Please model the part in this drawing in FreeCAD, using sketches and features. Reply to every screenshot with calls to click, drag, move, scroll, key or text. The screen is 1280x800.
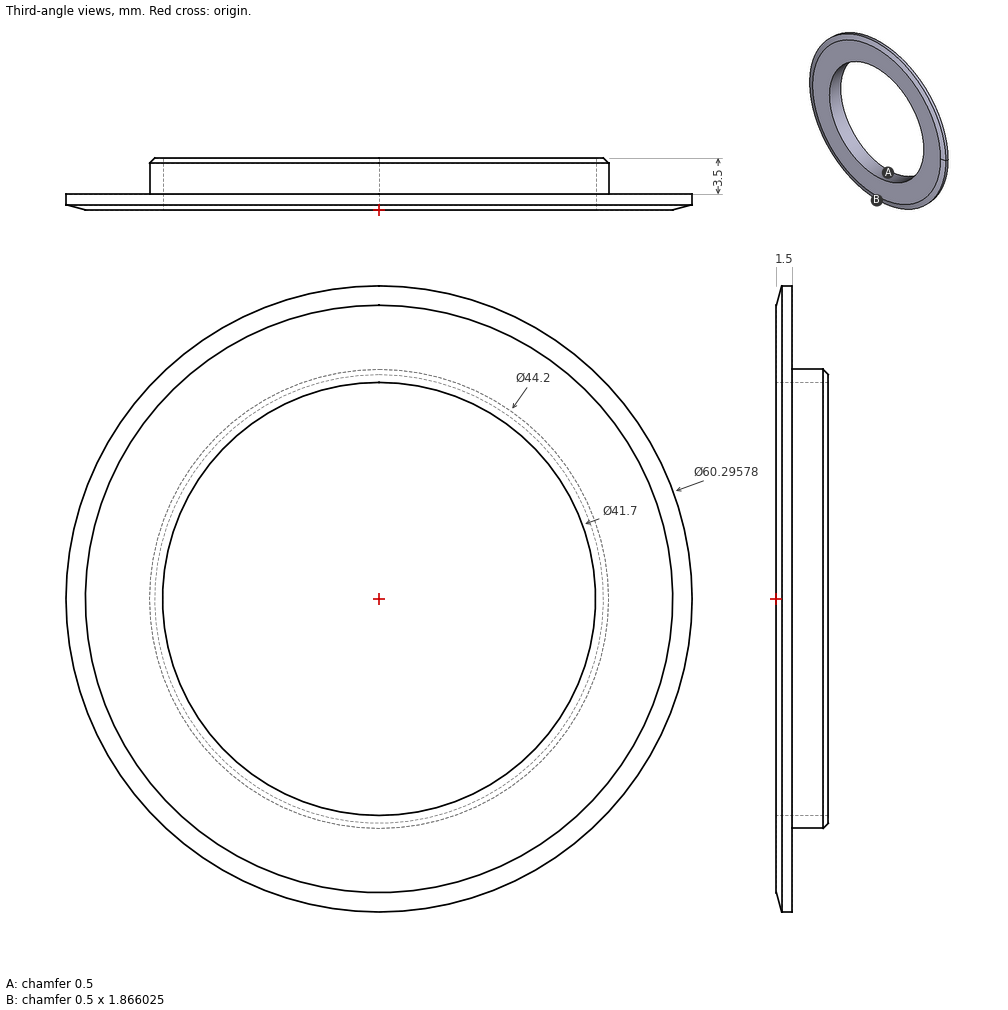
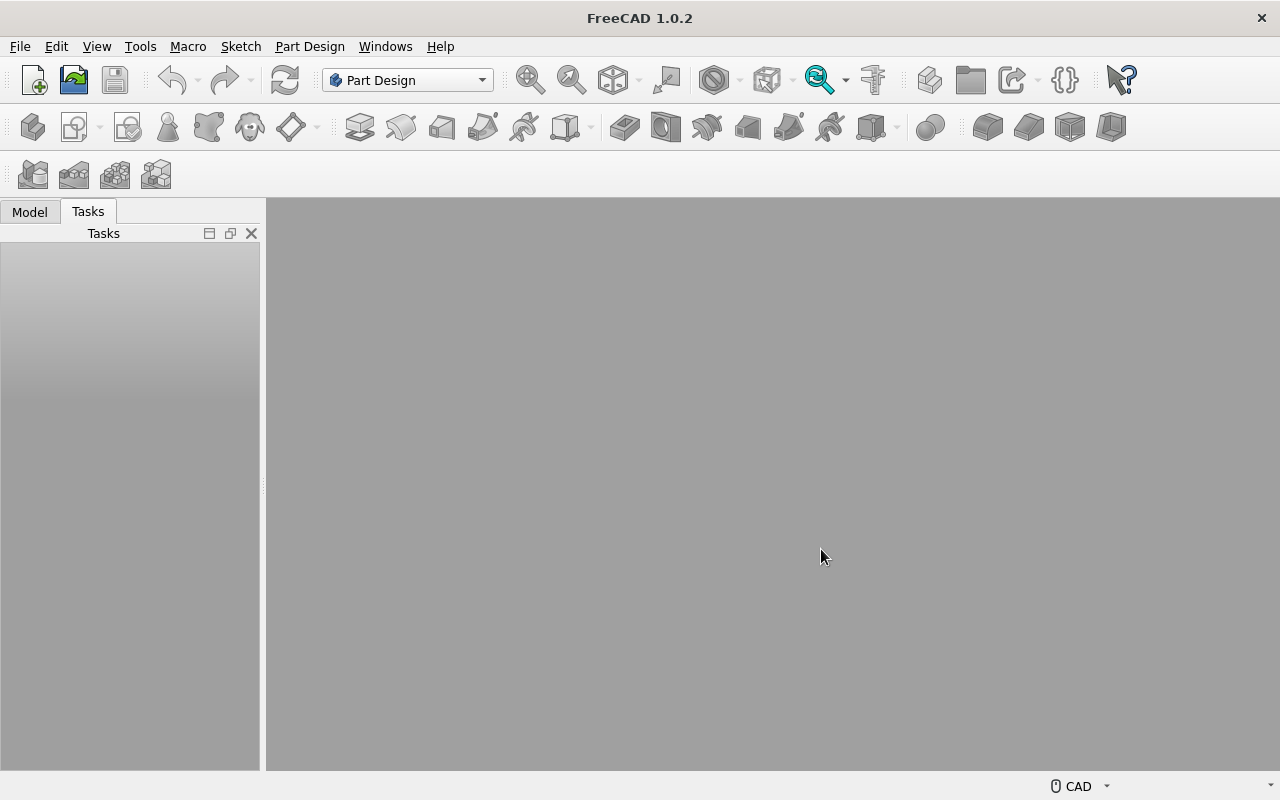
key(ctrl+n)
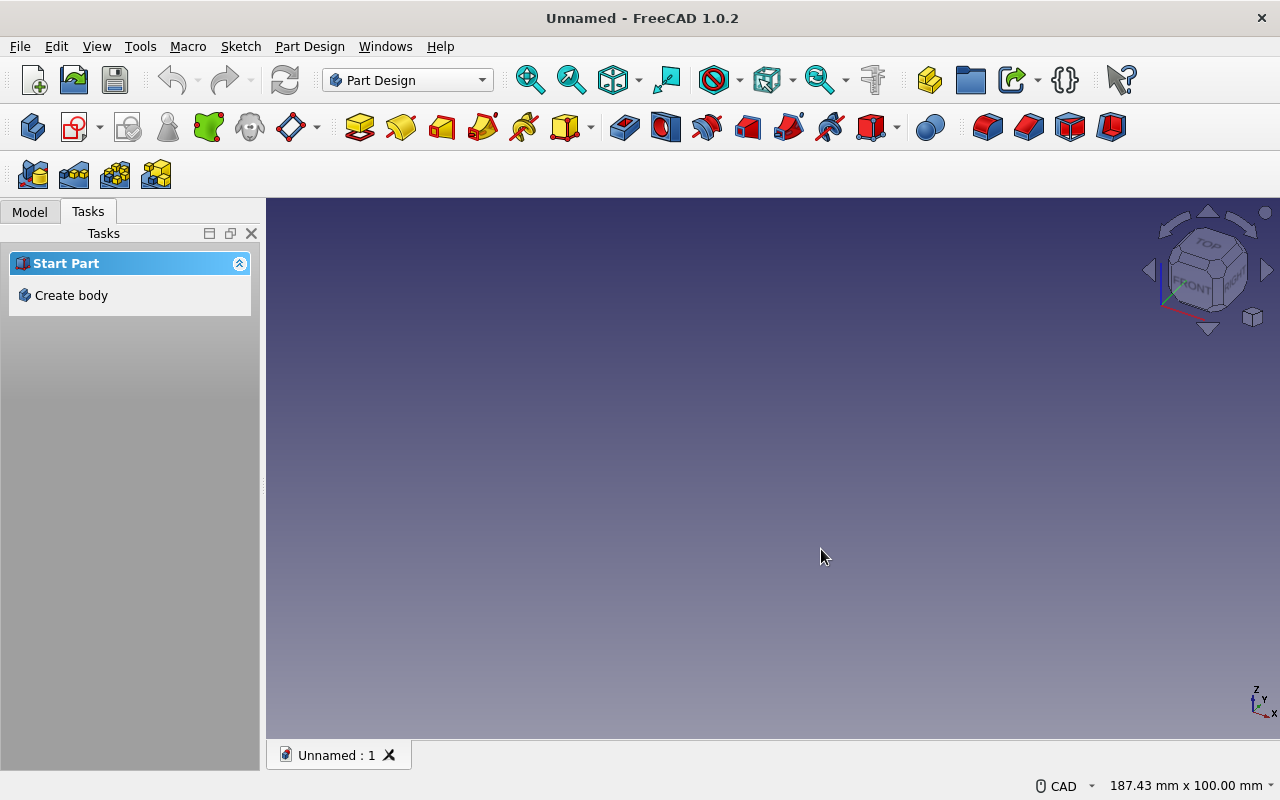
click(74, 128)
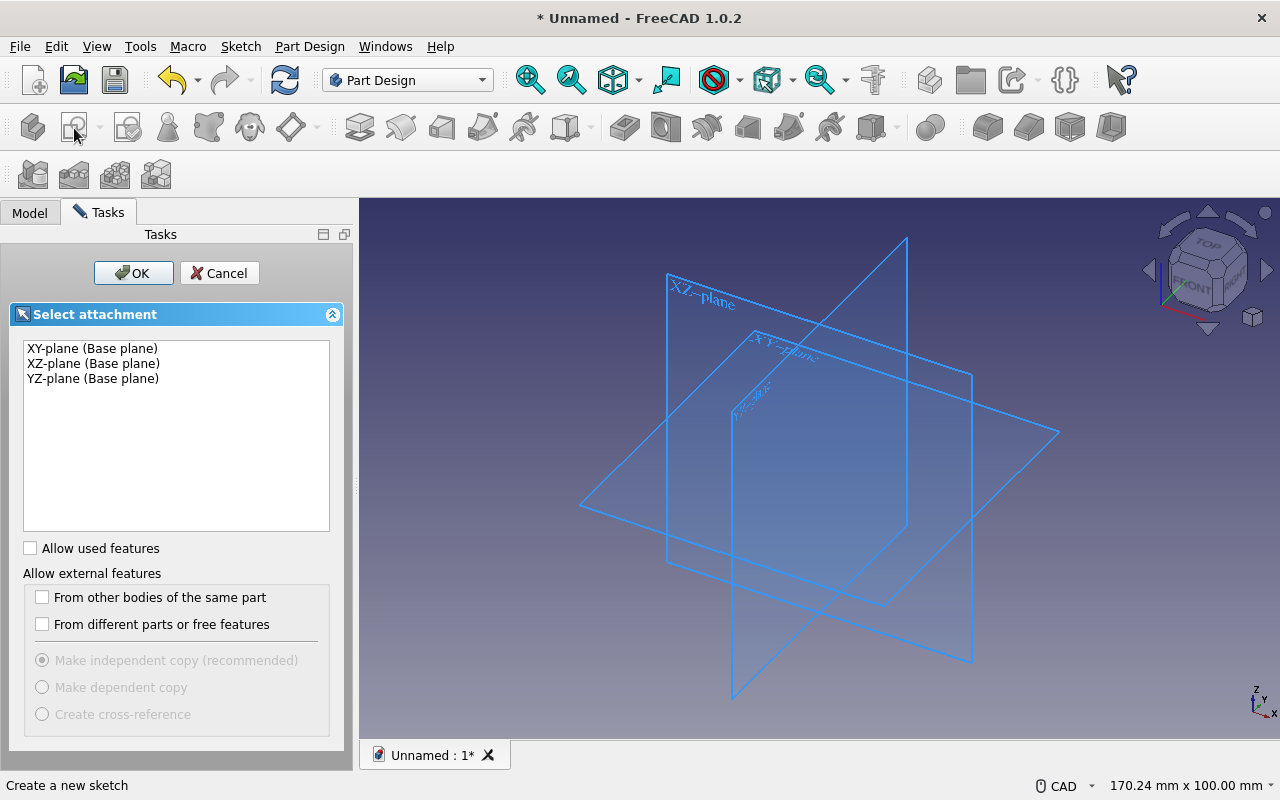
click(84, 364)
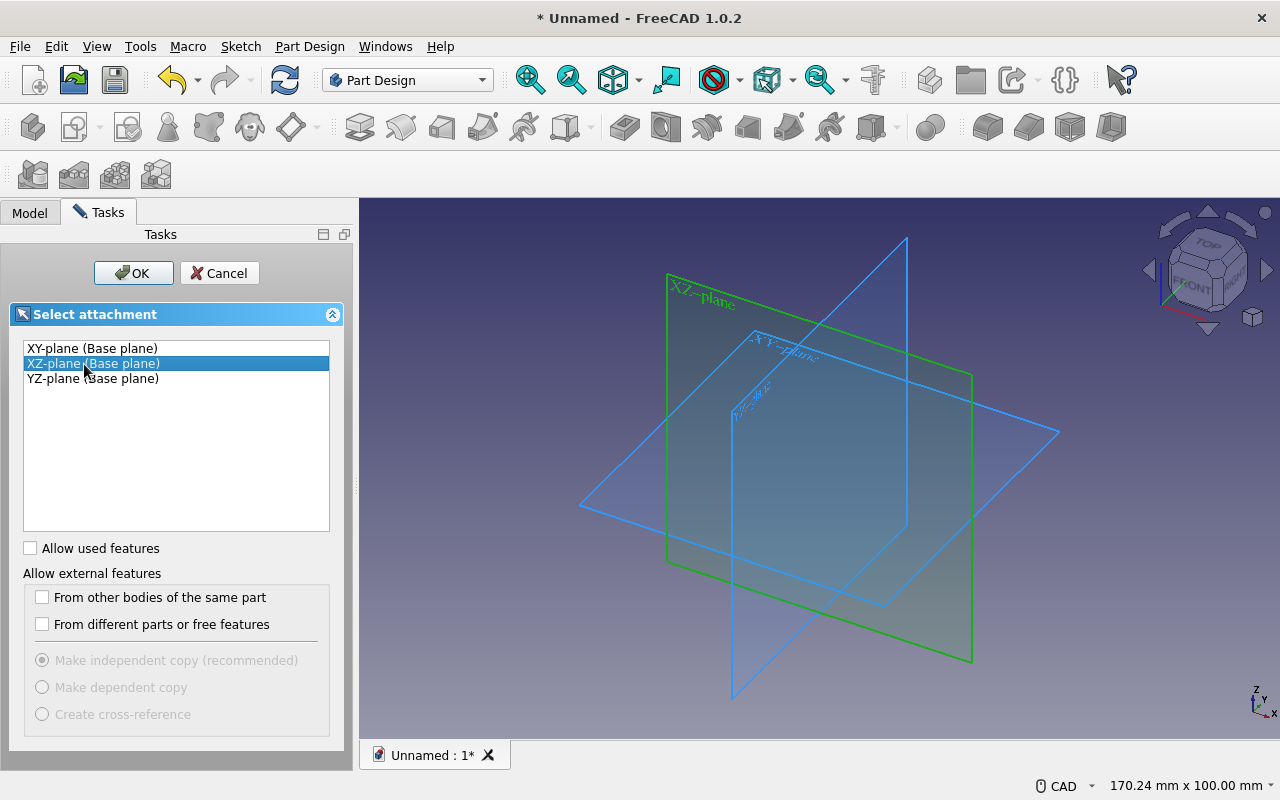
click(134, 273)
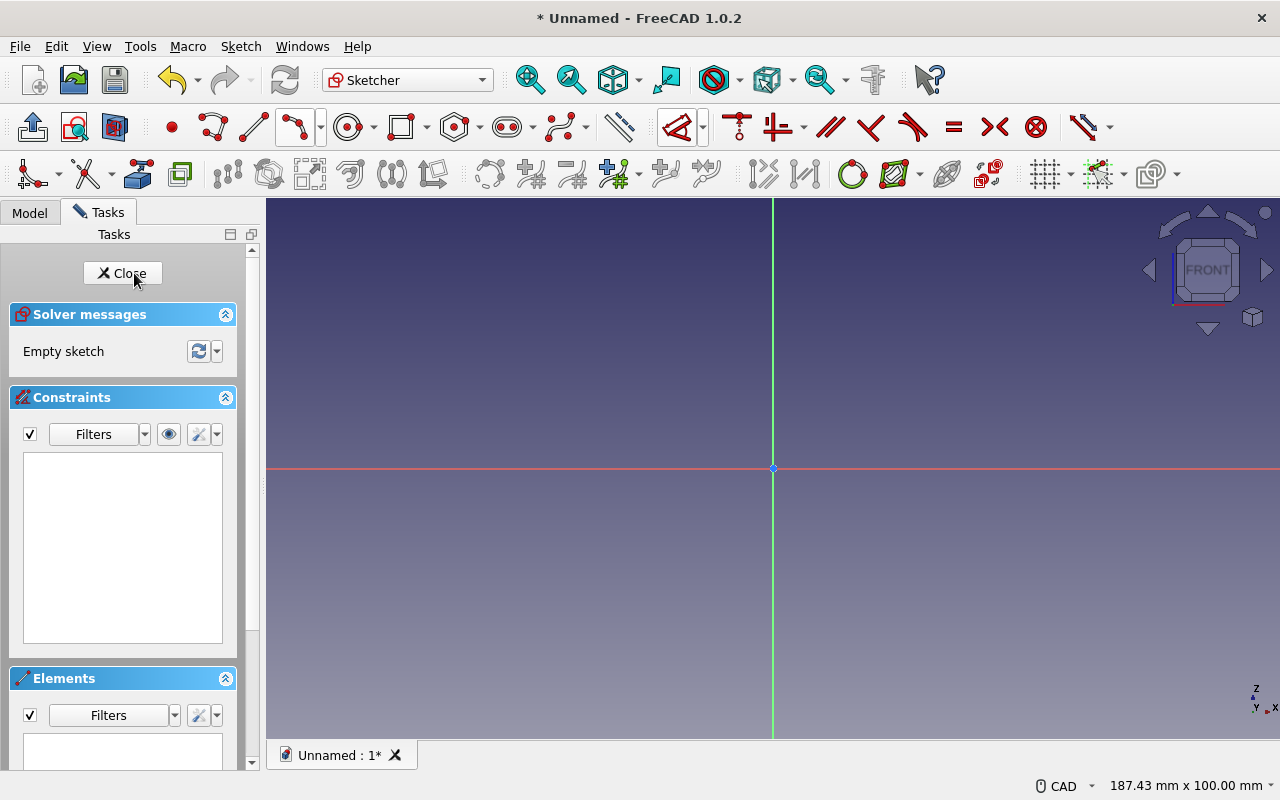
key(g)
key(c)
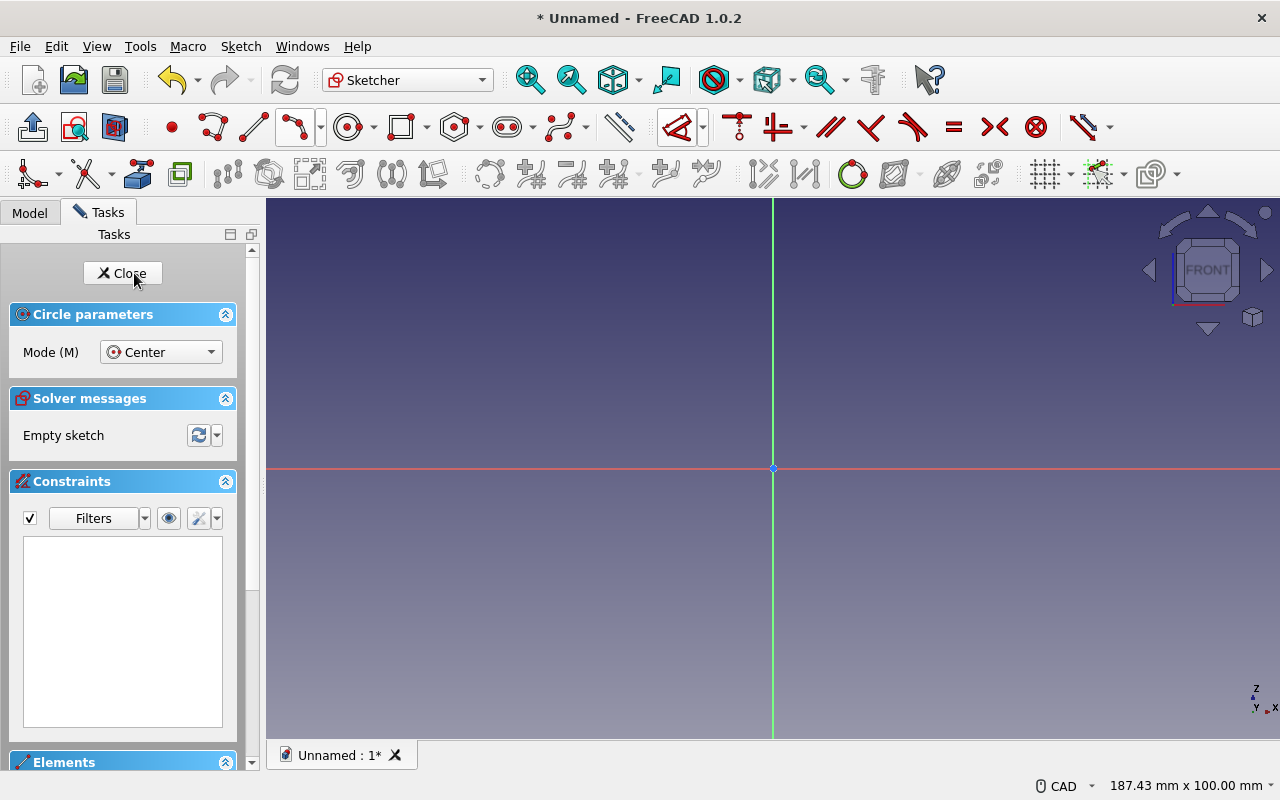
click(773, 468)
click(888, 353)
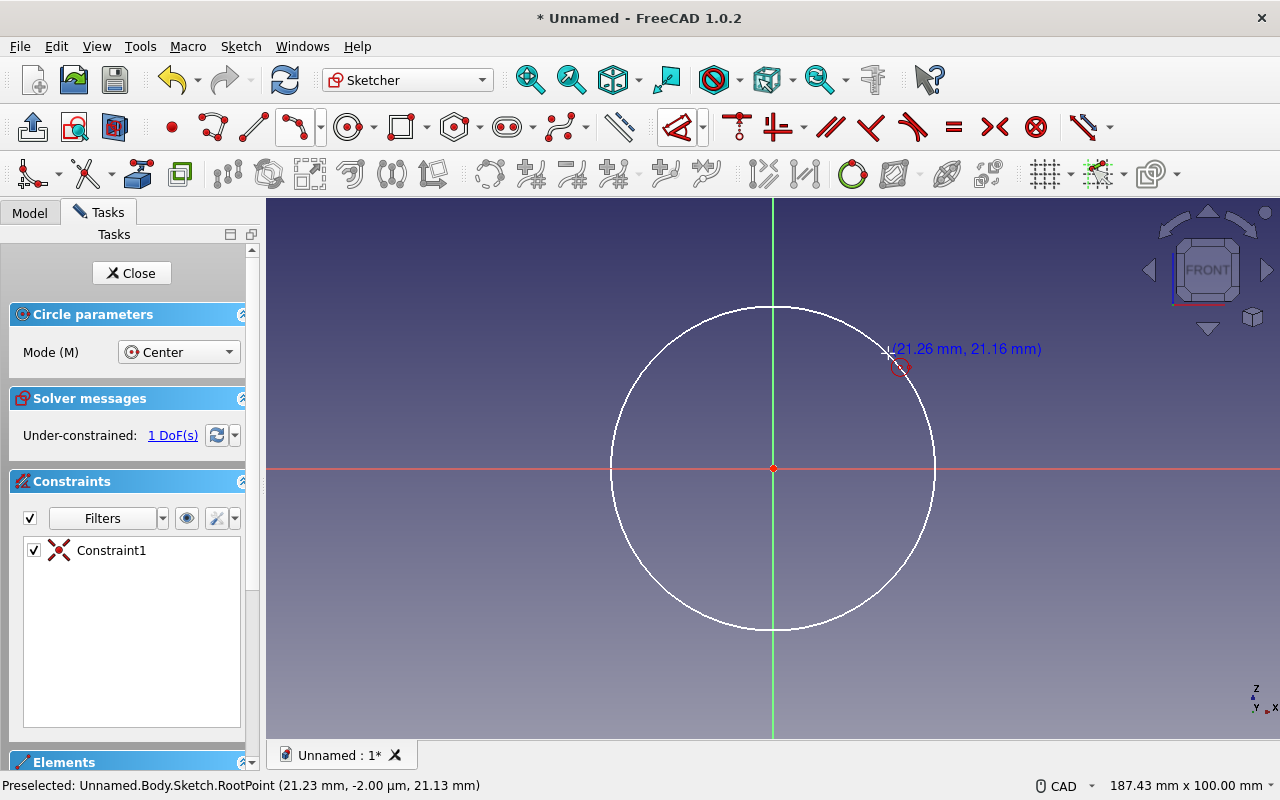
click(773, 468)
click(853, 389)
key(Escape)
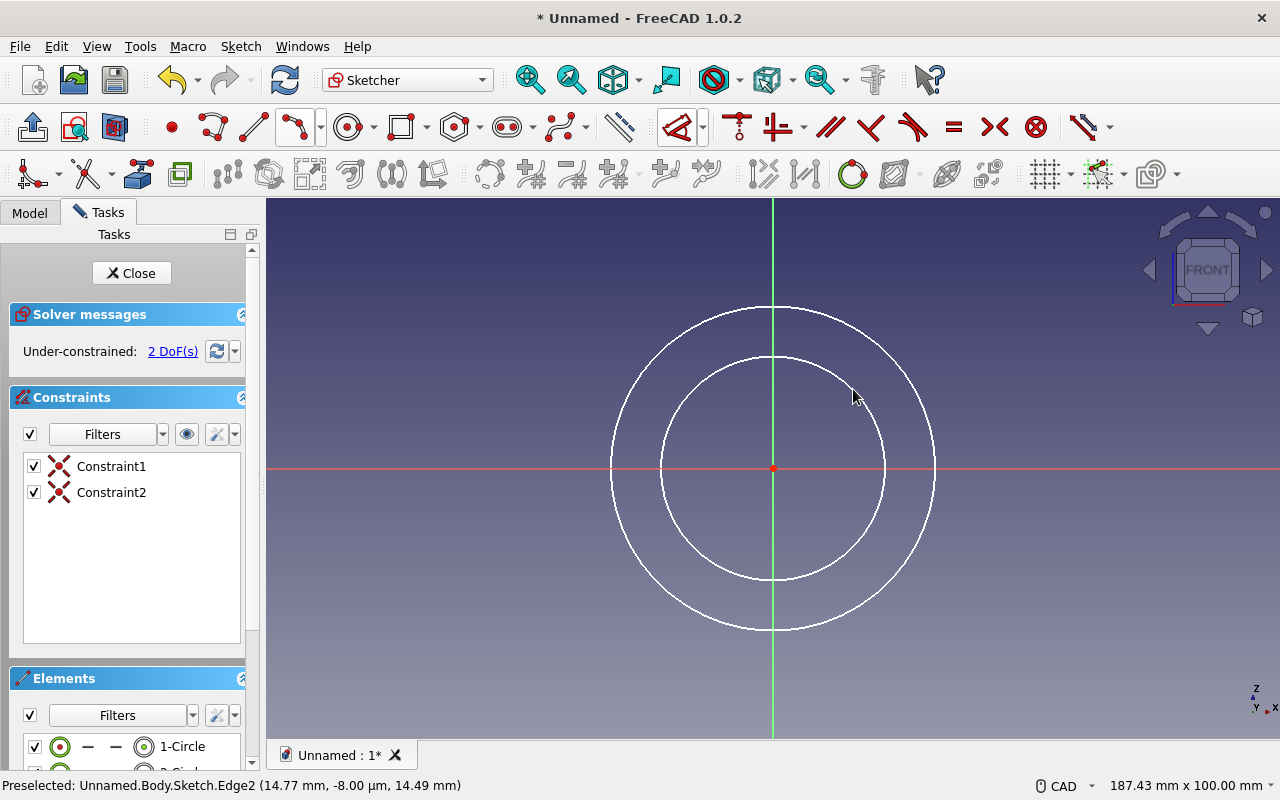
key(d)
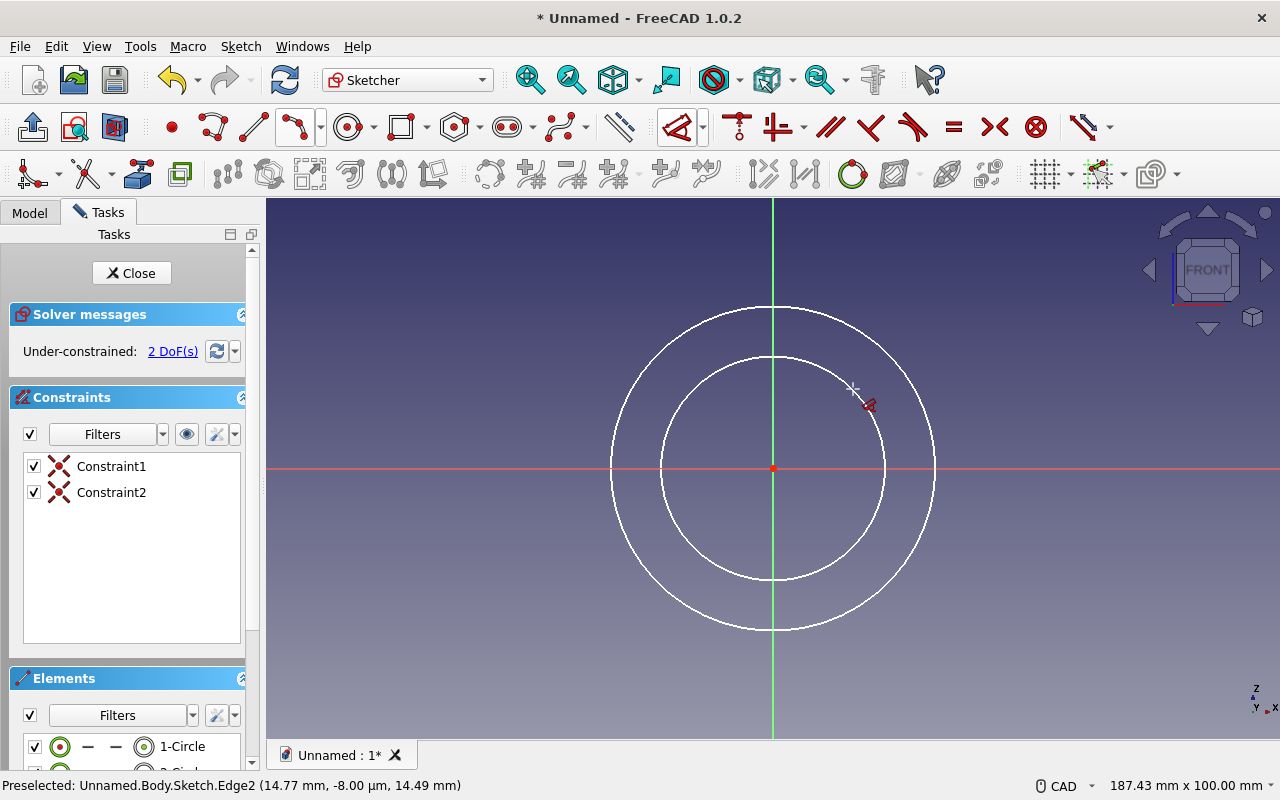
click(887, 353)
click(909, 330)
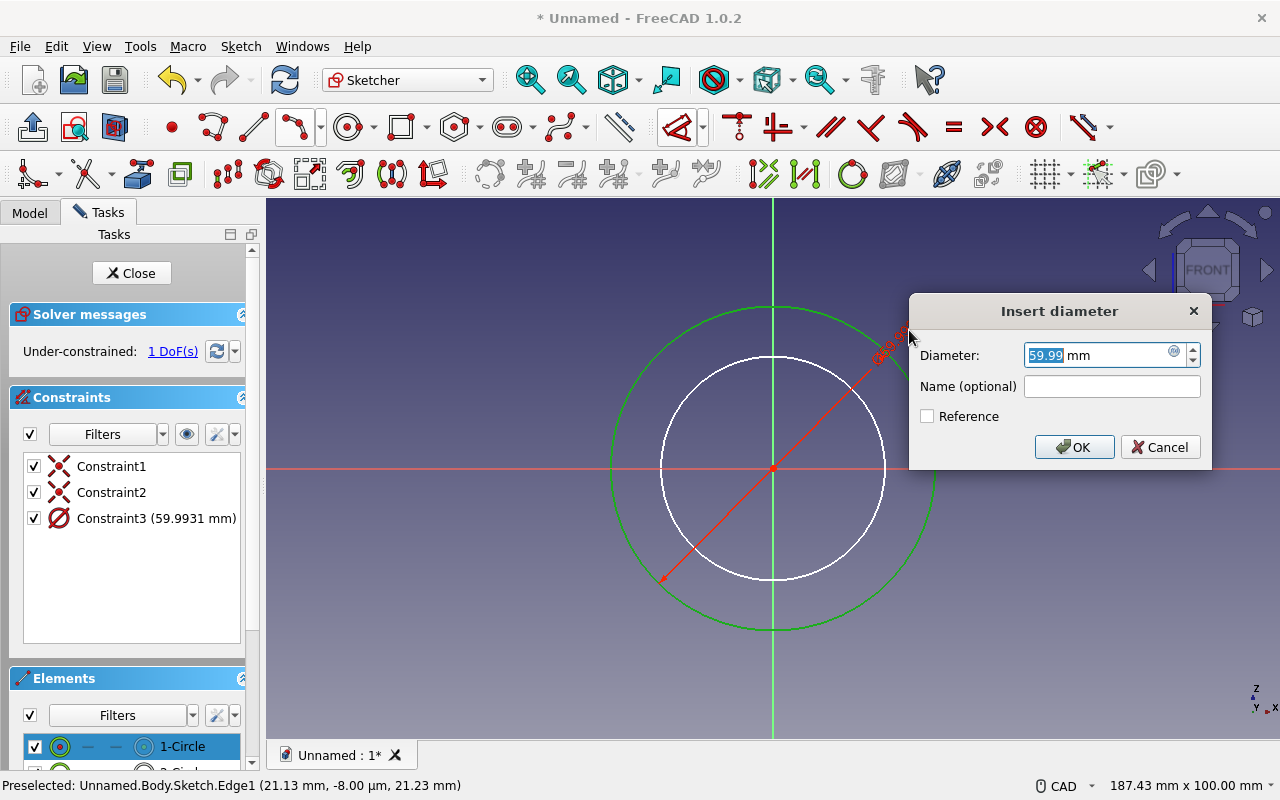
text(60.29578)
key(Return)